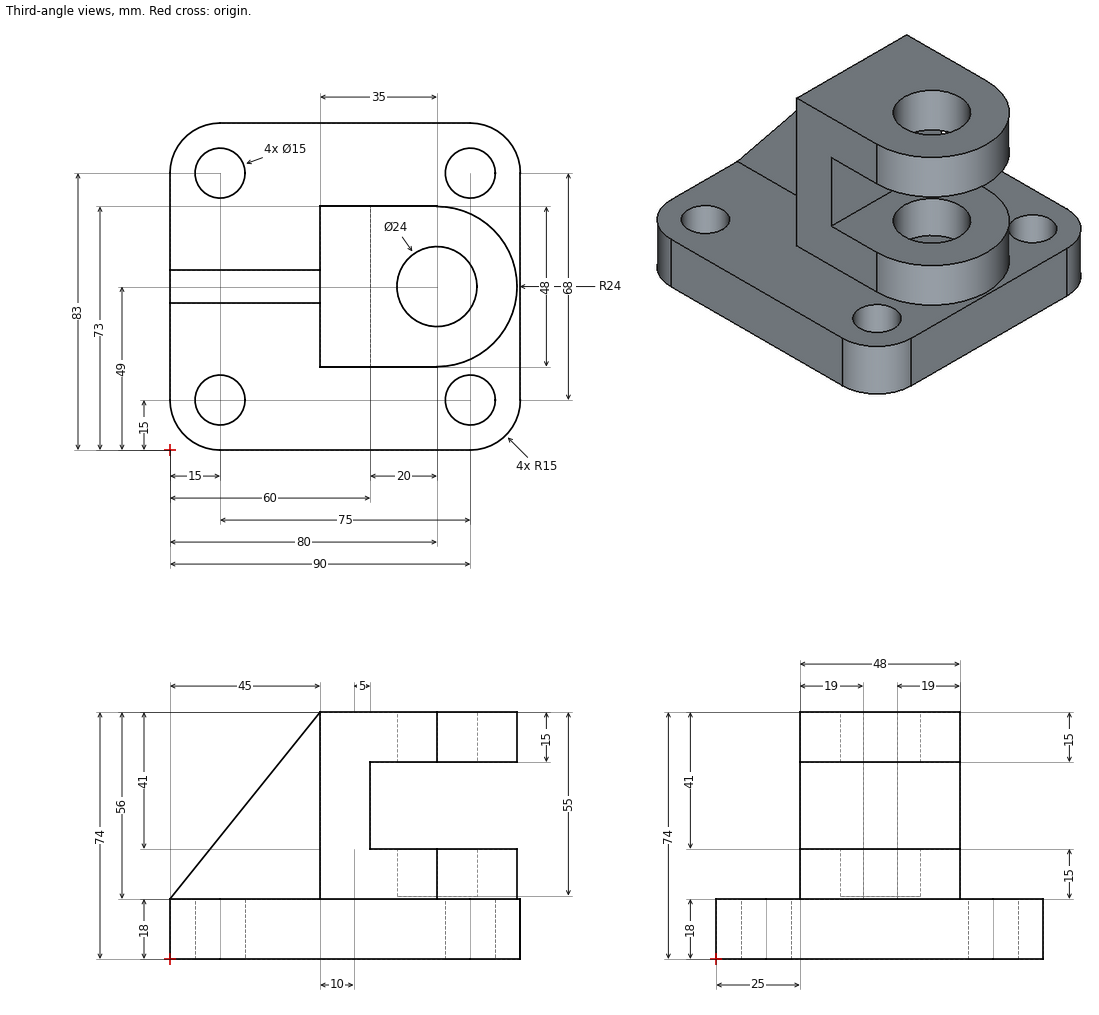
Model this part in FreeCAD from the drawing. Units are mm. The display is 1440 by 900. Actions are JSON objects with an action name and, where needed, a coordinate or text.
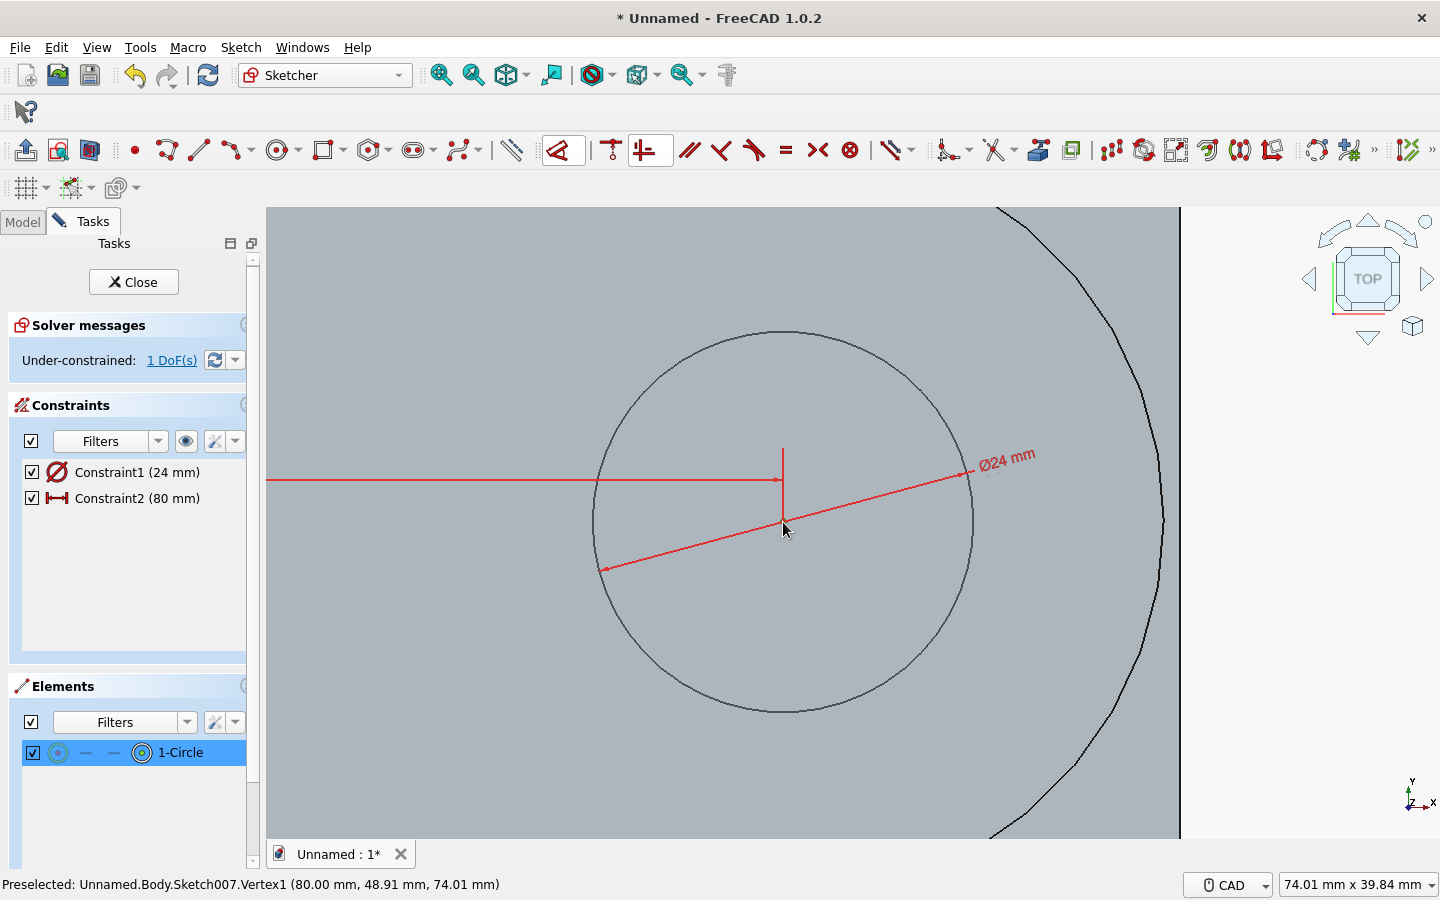
{"action": "left_click", "coordinate": [580, 150]}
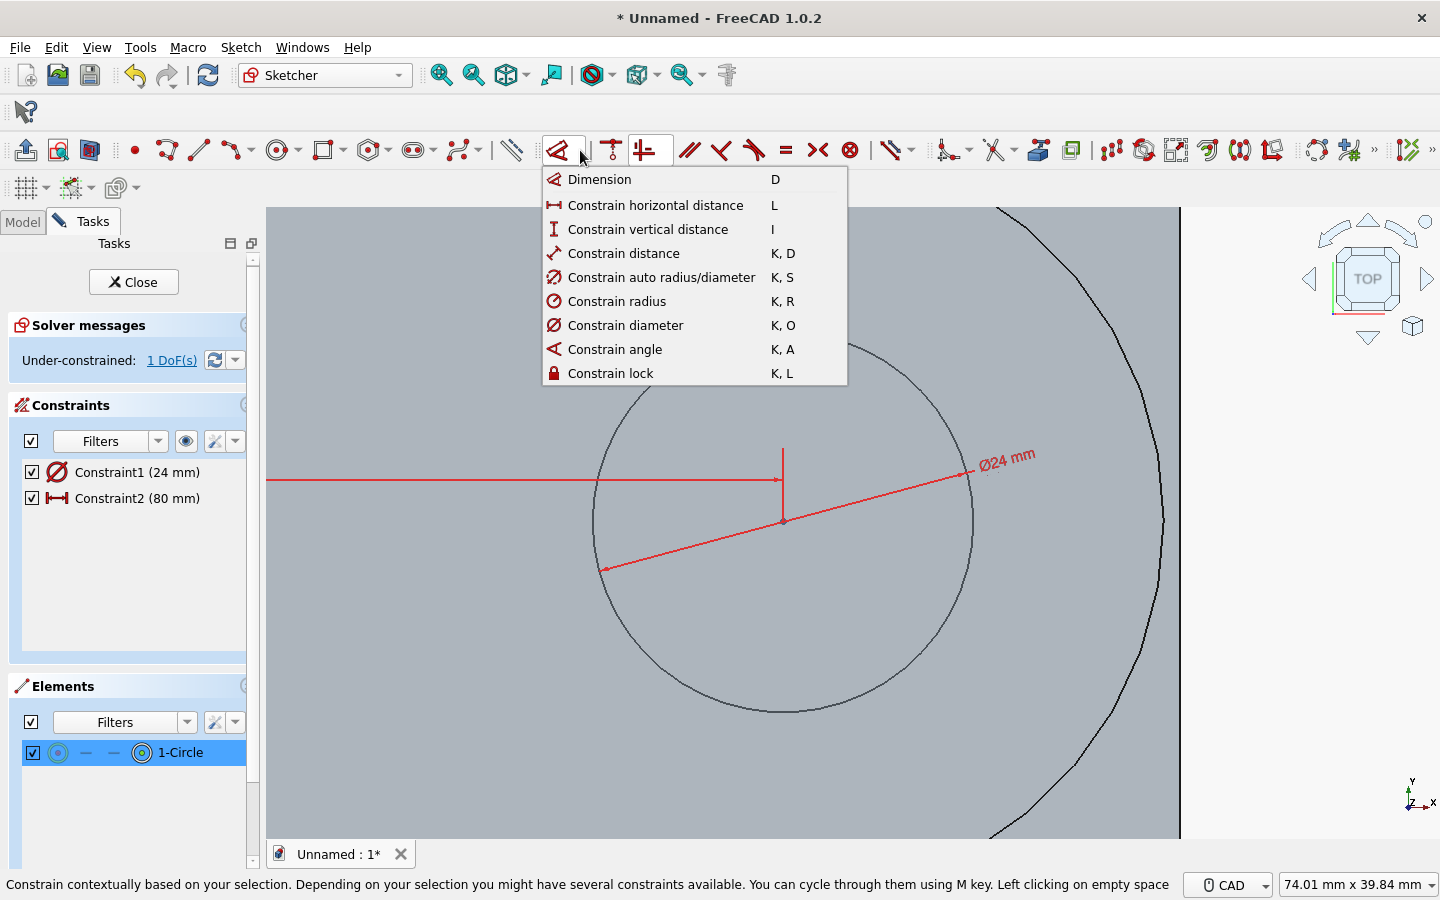
{"action": "left_click", "coordinate": [695, 229]}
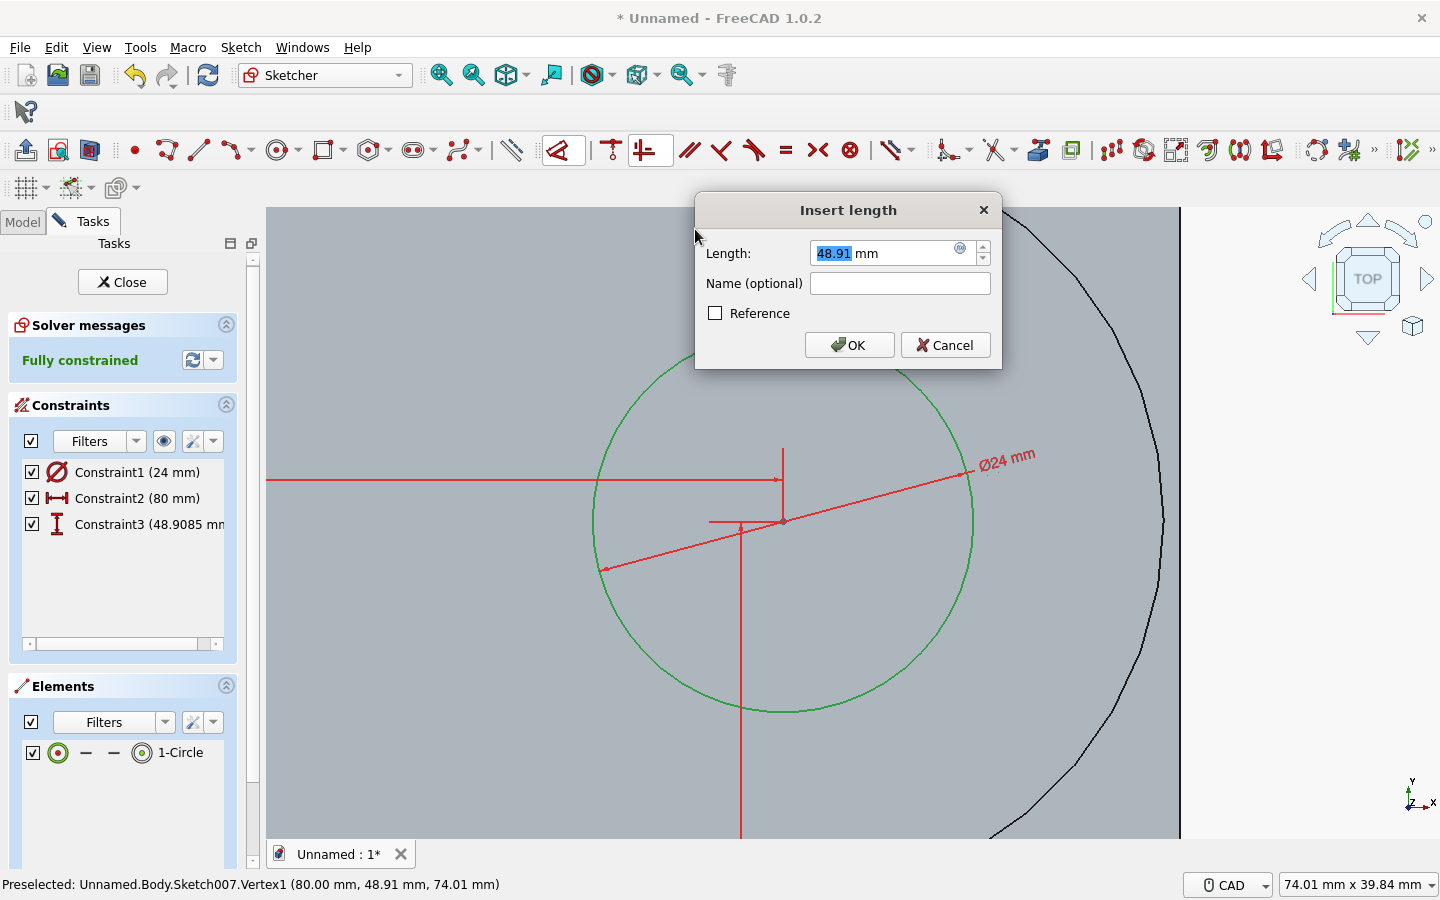
{"action": "type", "text": "49"}
{"action": "key", "text": "Return"}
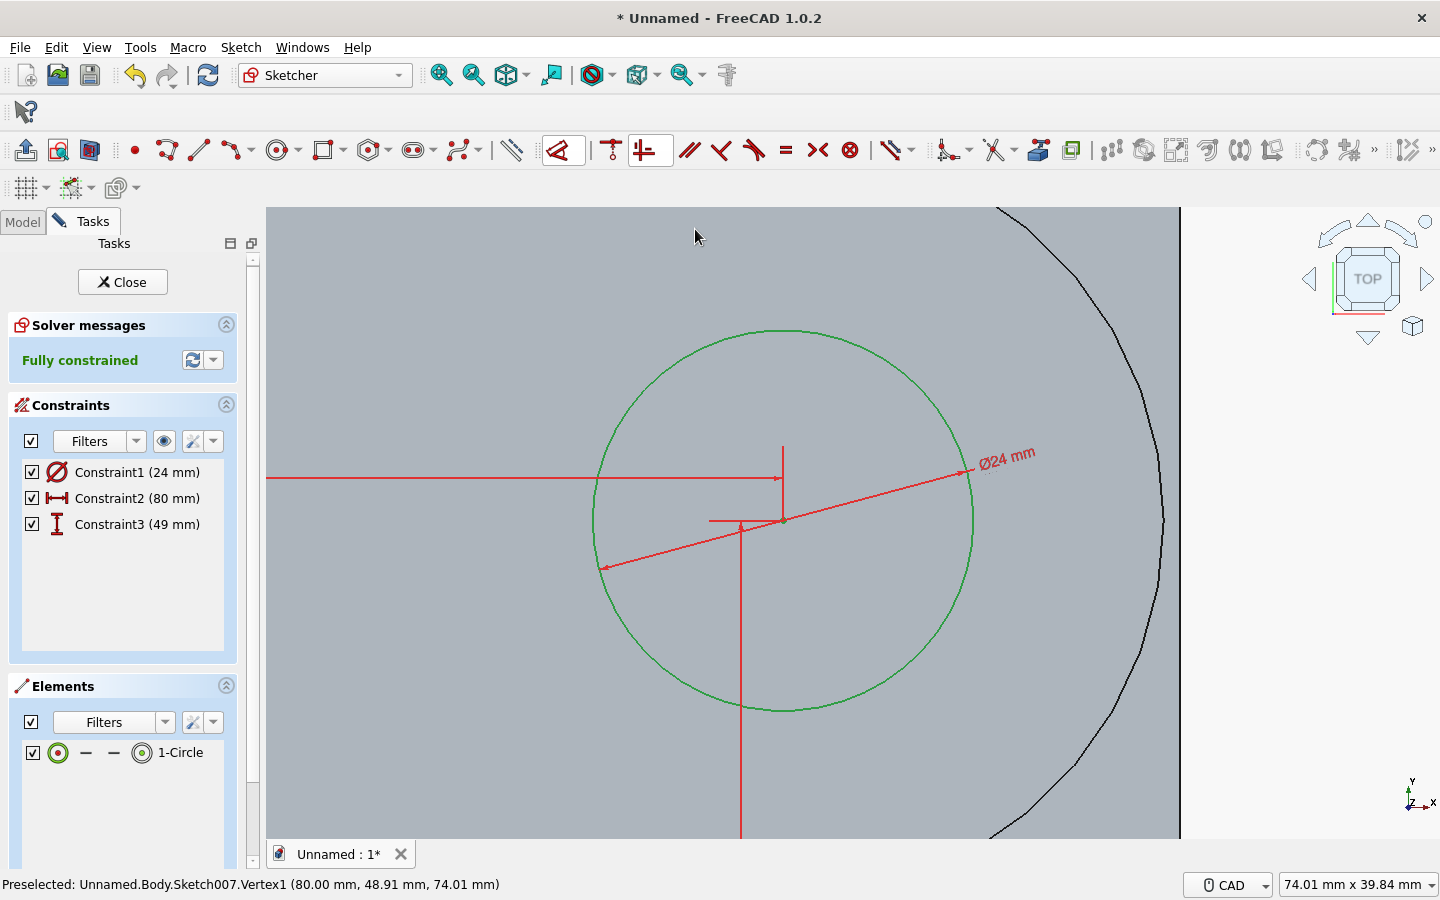
{"action": "left_click", "coordinate": [123, 282]}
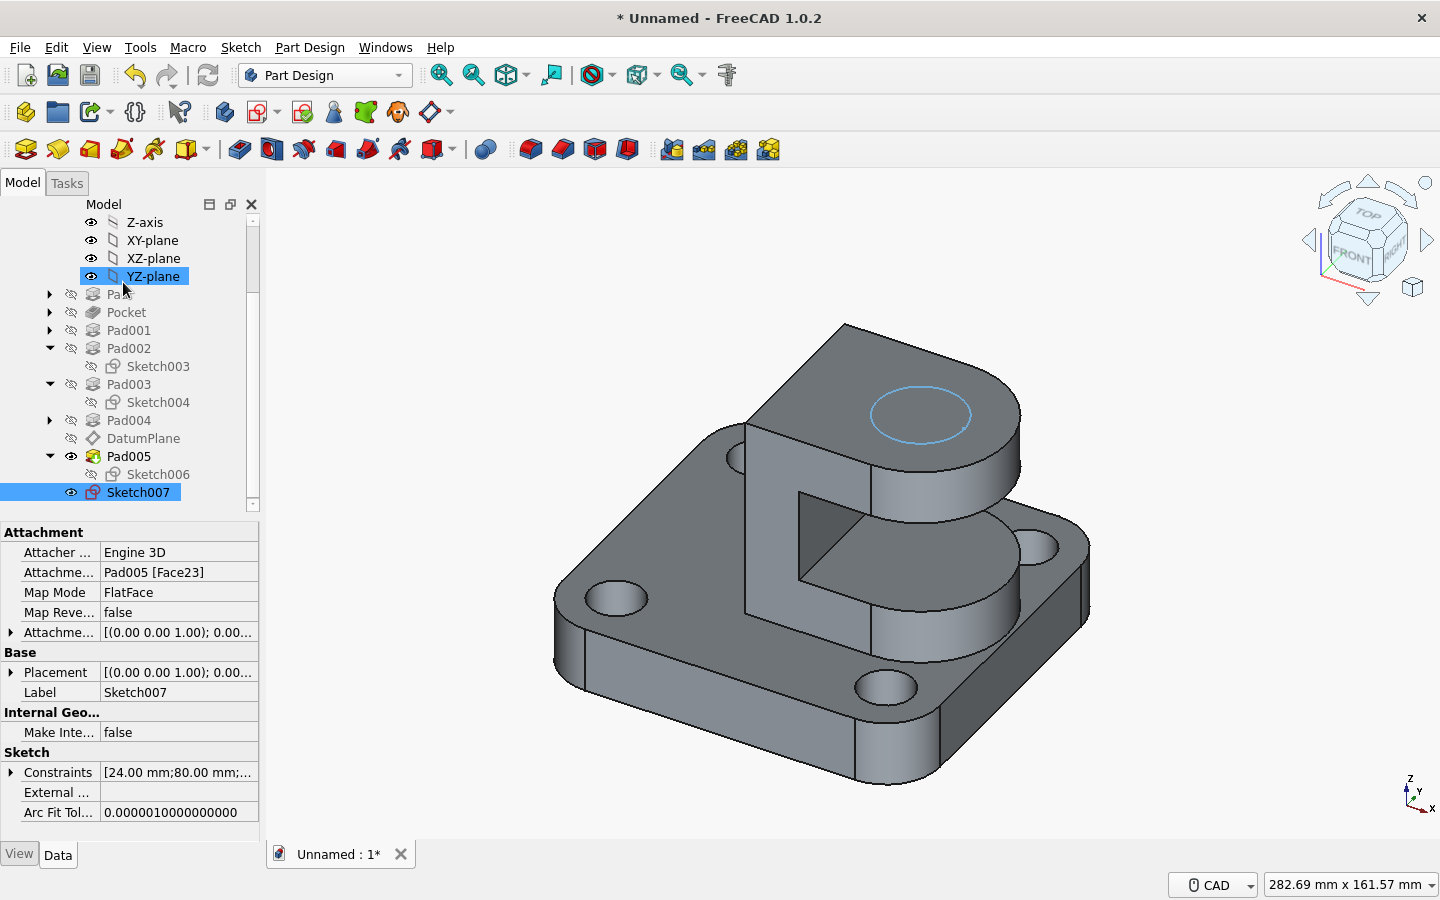
{"action": "left_click", "coordinate": [240, 150]}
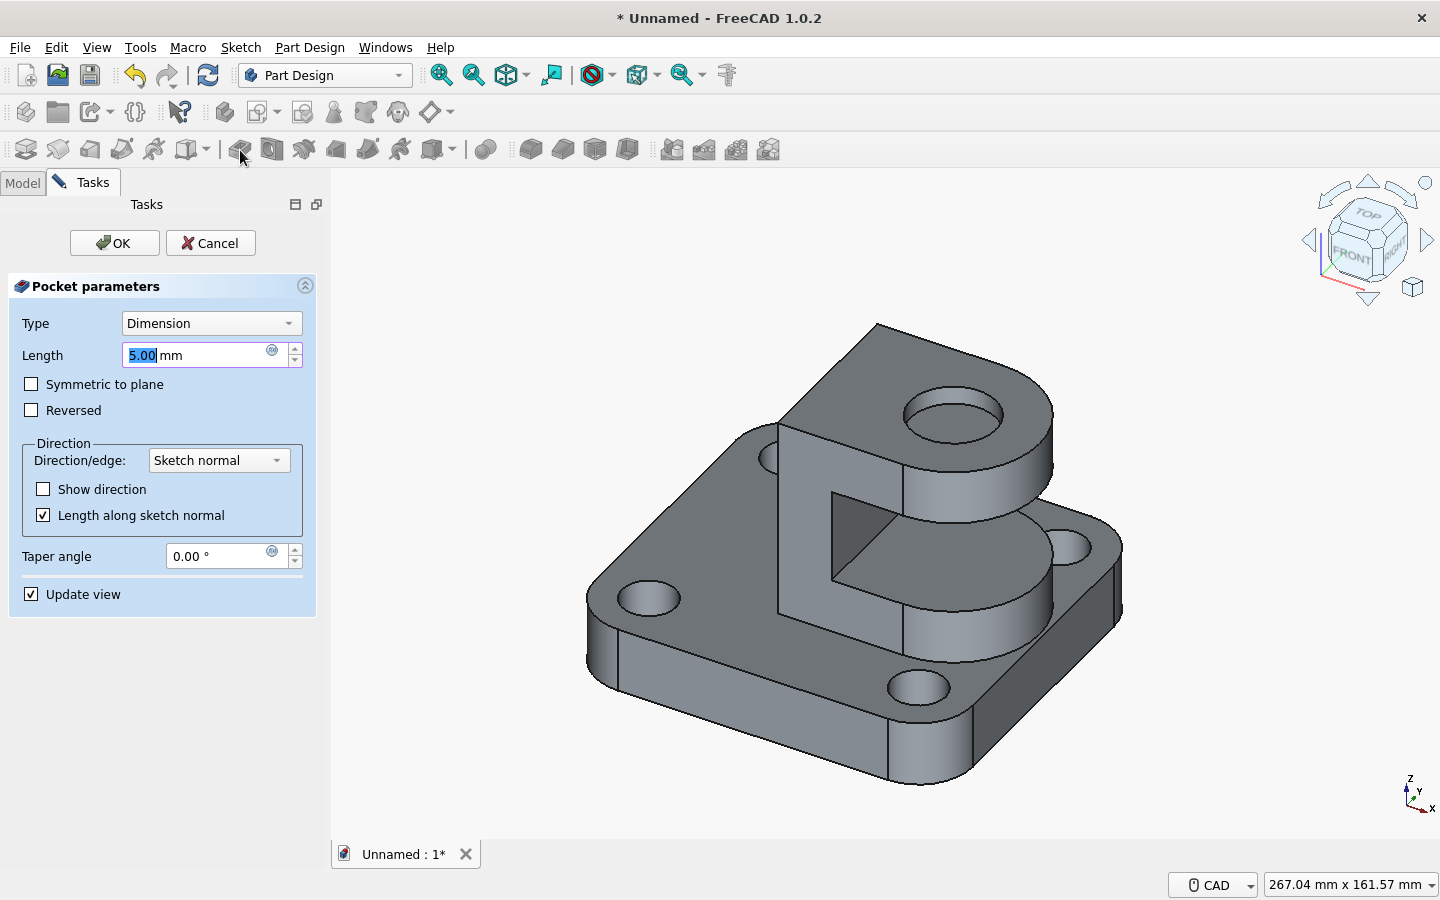
{"action": "type", "text": "55"}
{"action": "key", "text": "Tab"}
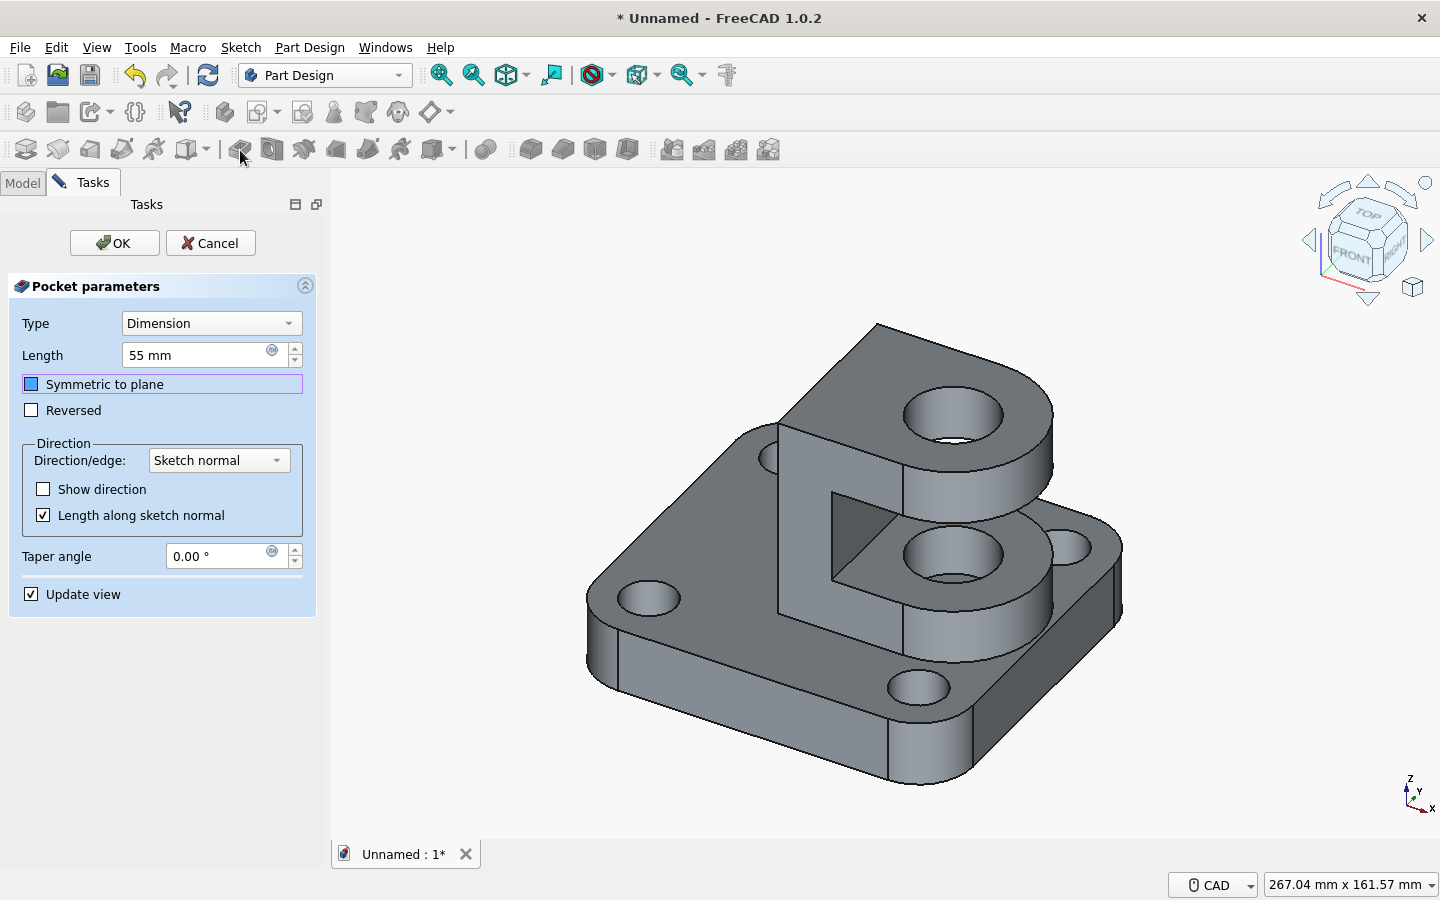
{"action": "left_click", "coordinate": [115, 243]}